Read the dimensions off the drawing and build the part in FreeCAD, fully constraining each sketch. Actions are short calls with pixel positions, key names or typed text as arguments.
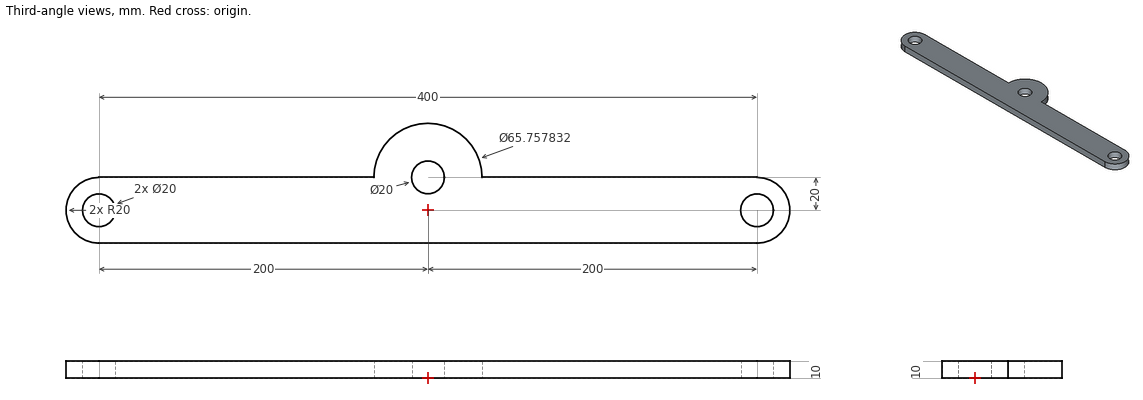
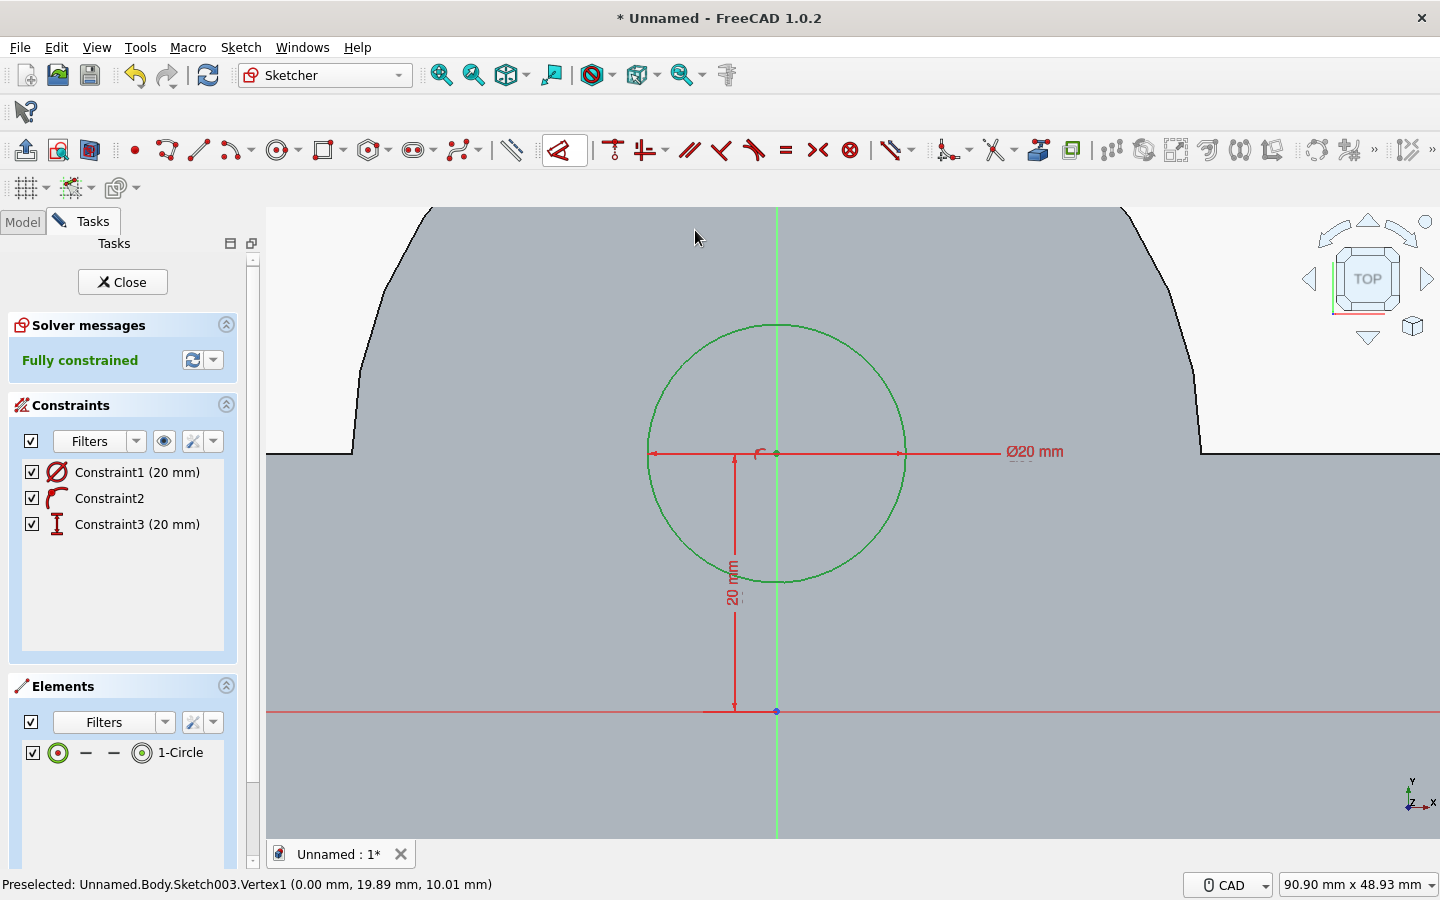
click(123, 282)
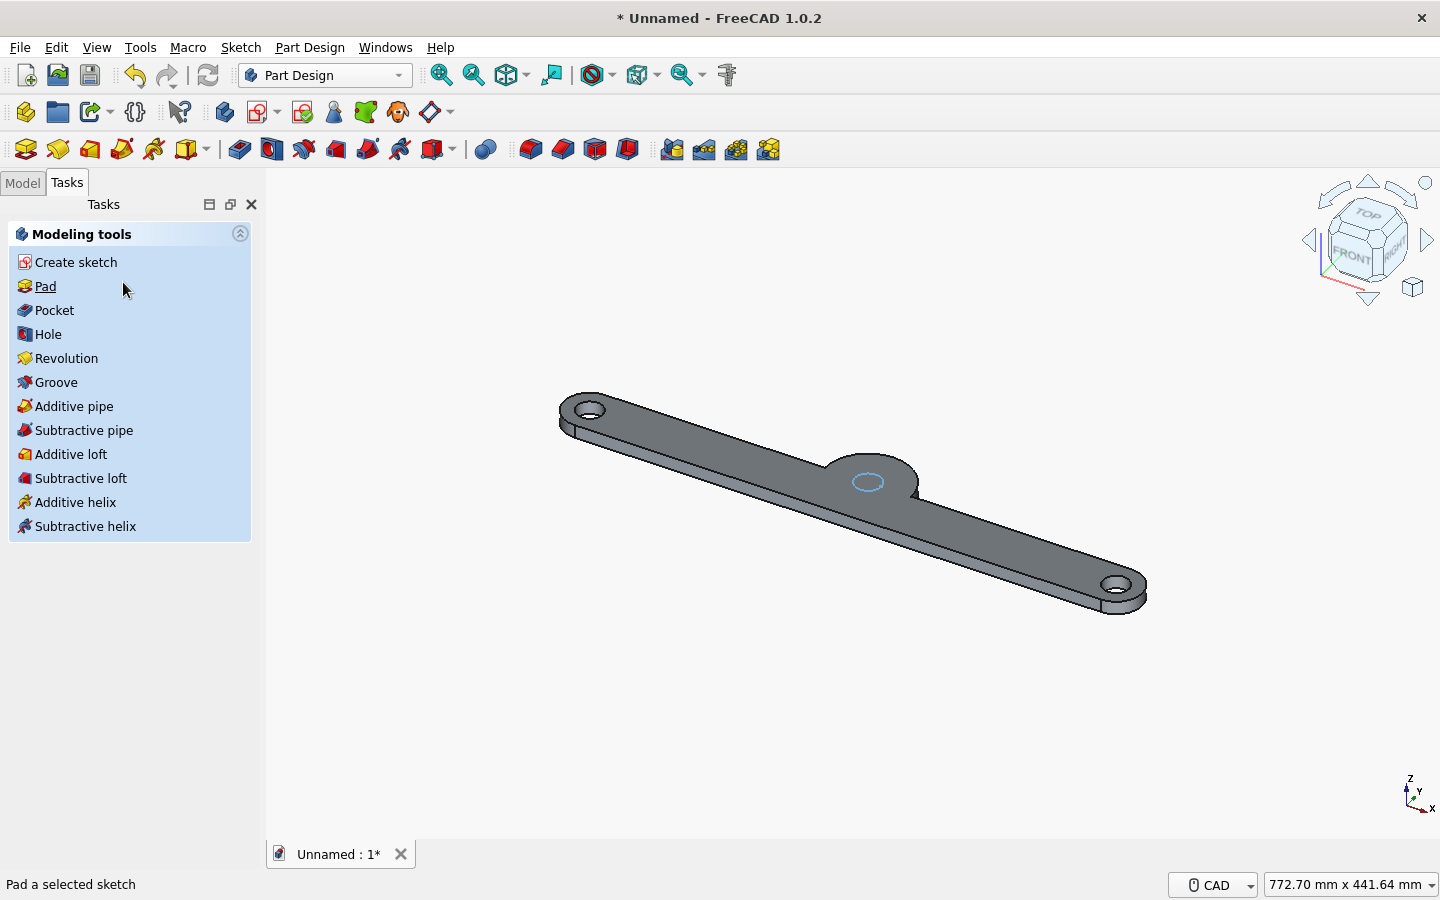
click(240, 150)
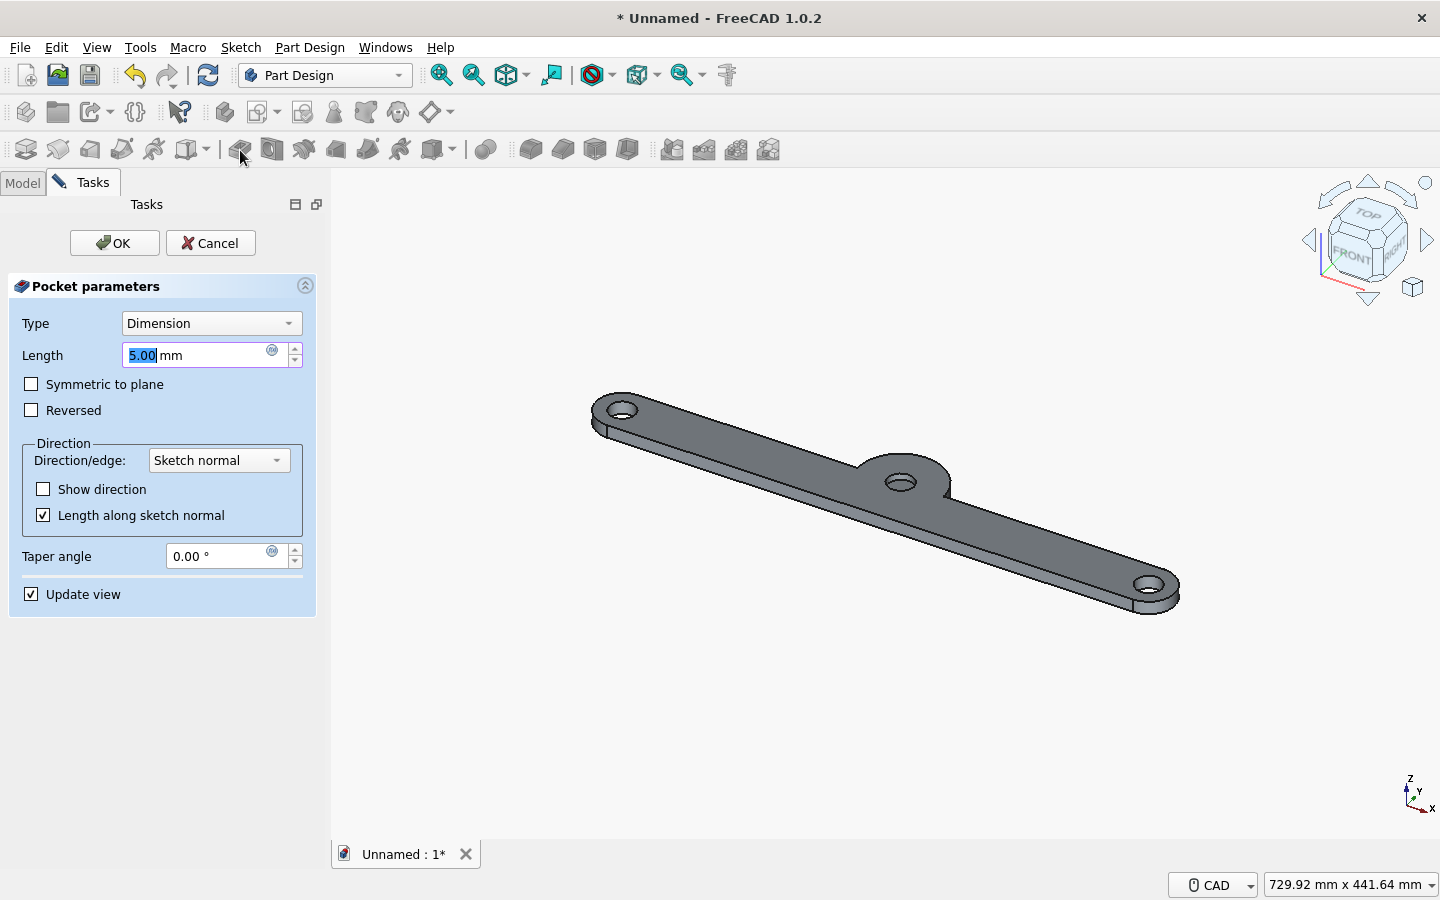
click(212, 324)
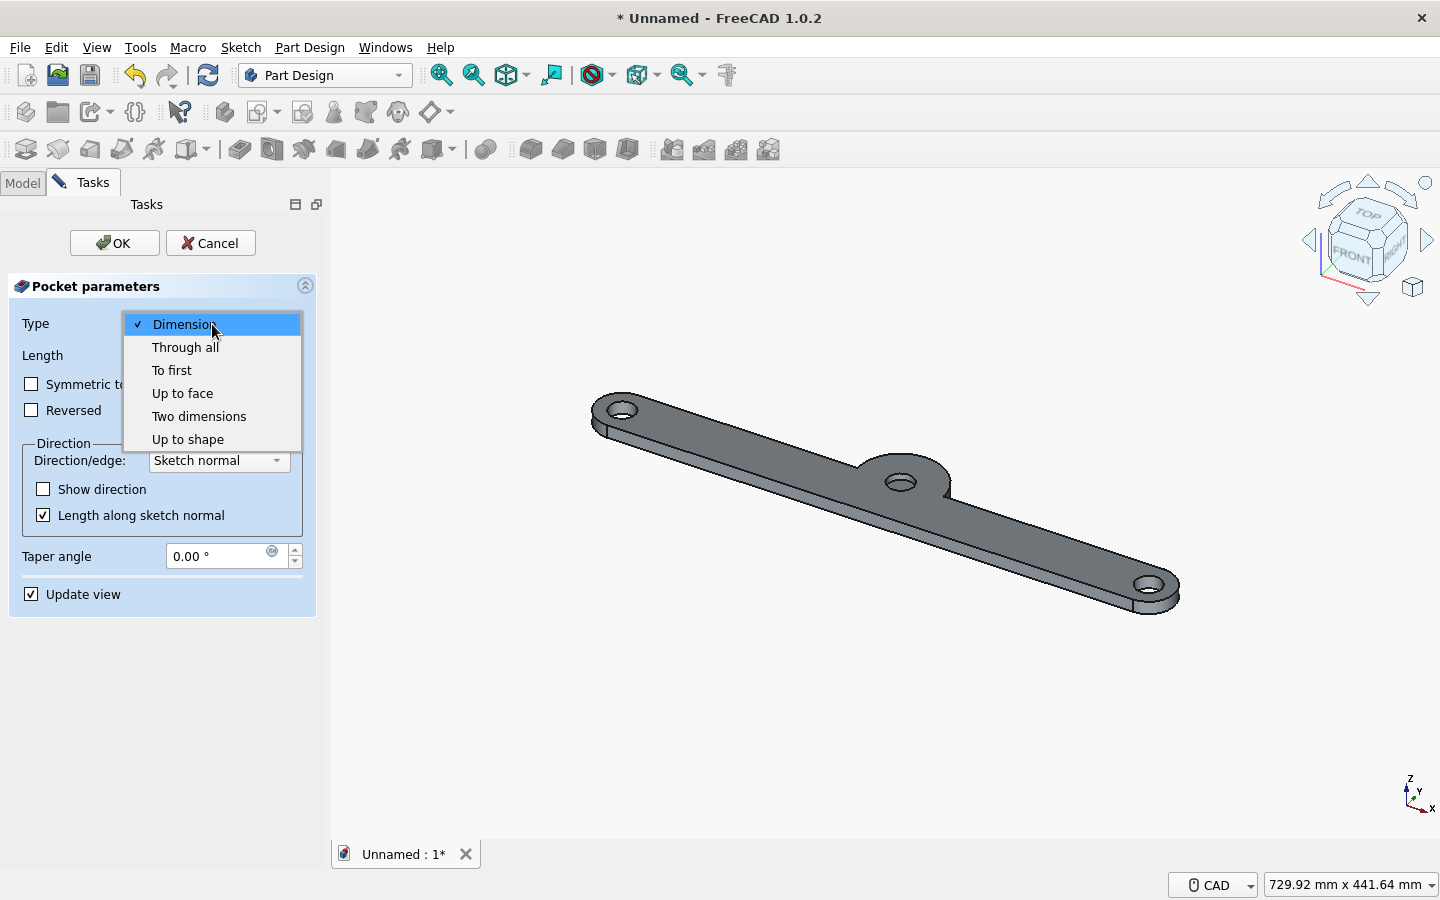
click(212, 348)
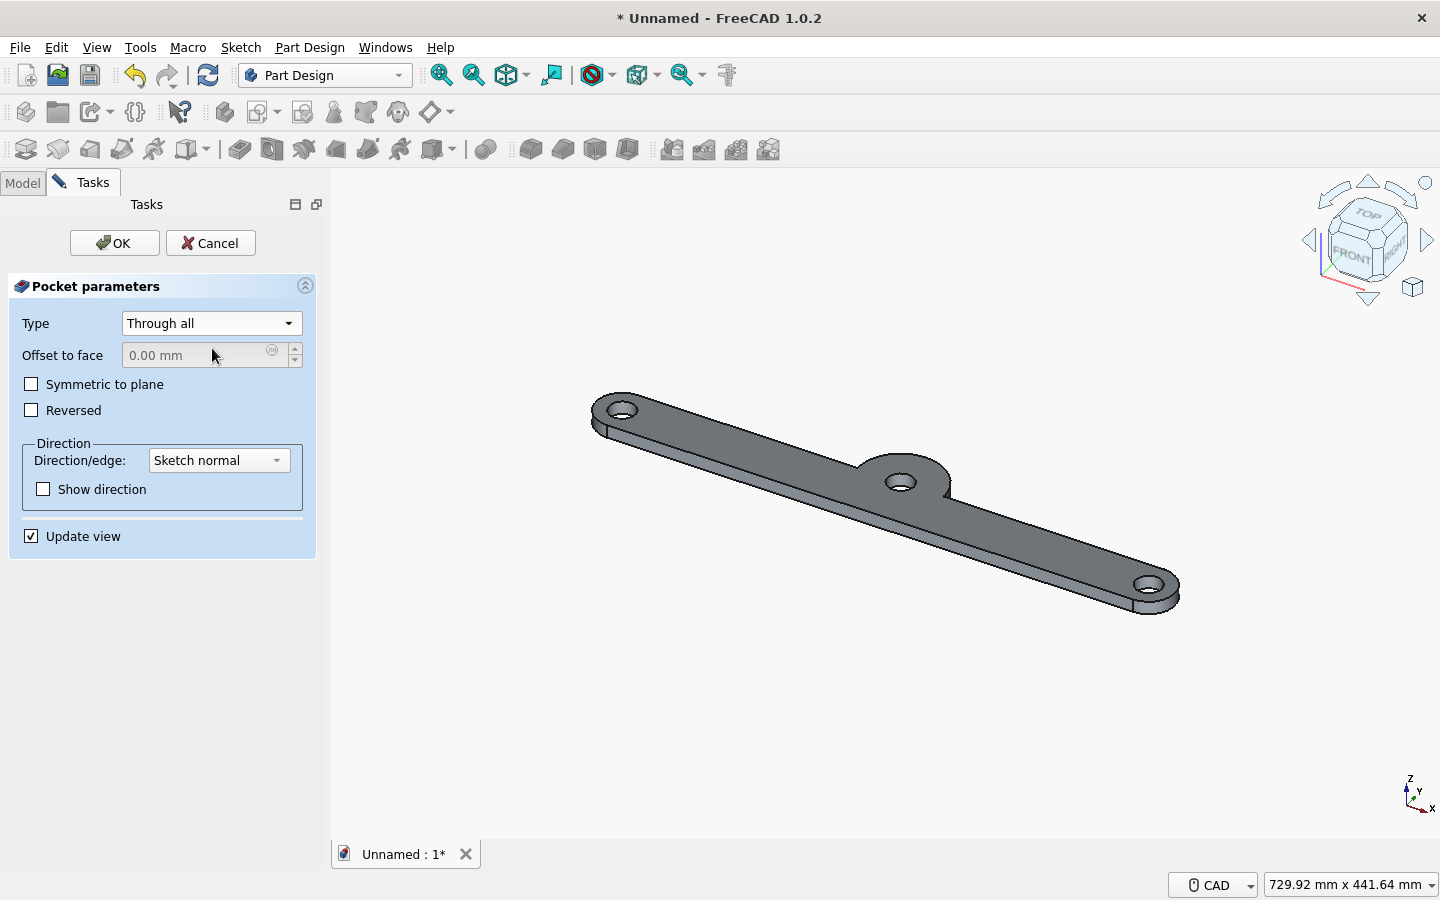
click(115, 243)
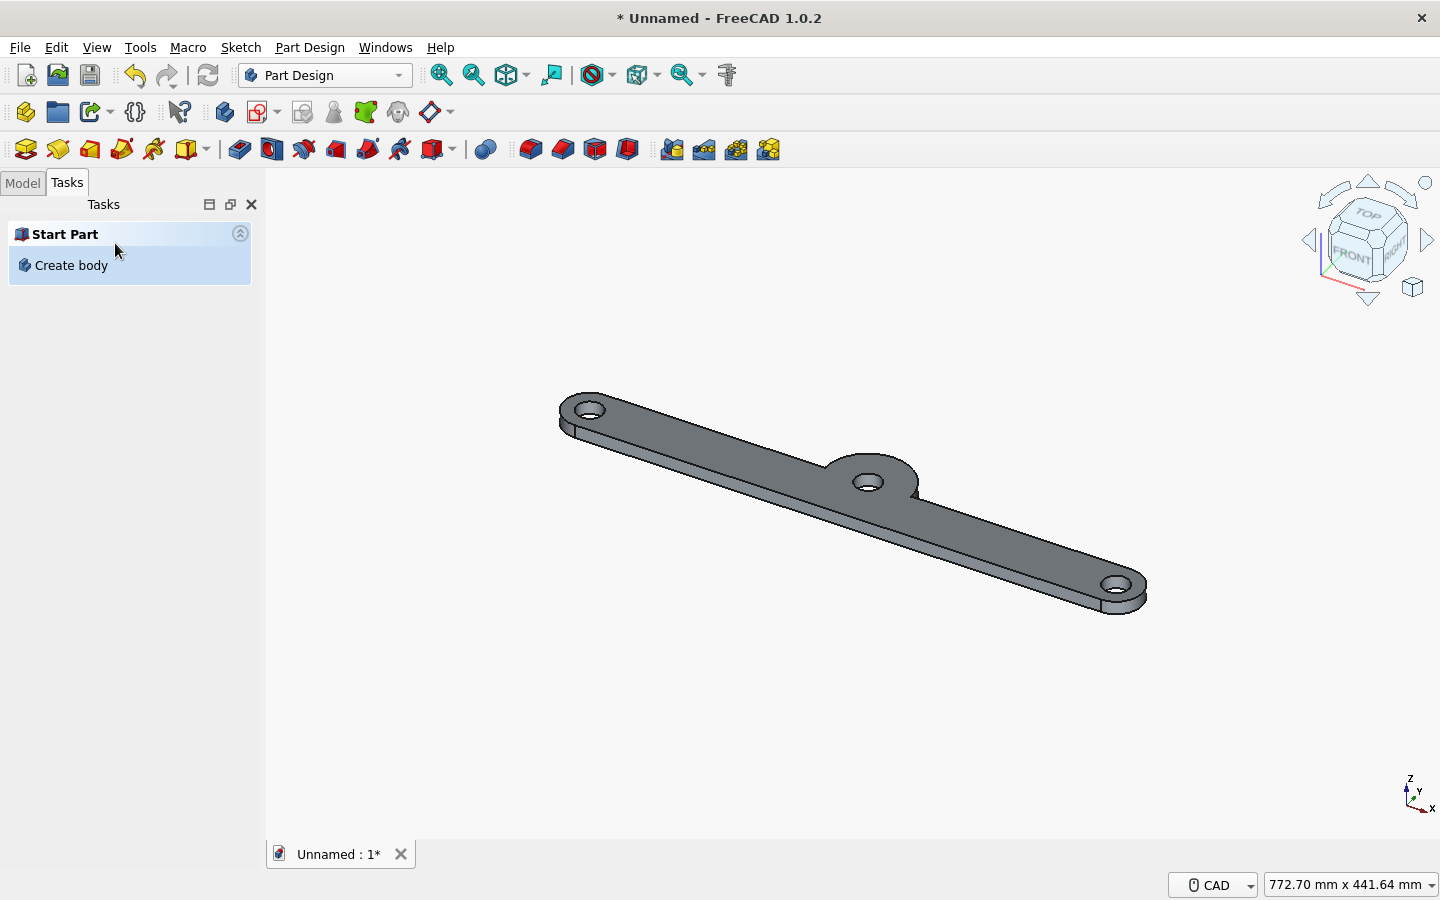
key(0)